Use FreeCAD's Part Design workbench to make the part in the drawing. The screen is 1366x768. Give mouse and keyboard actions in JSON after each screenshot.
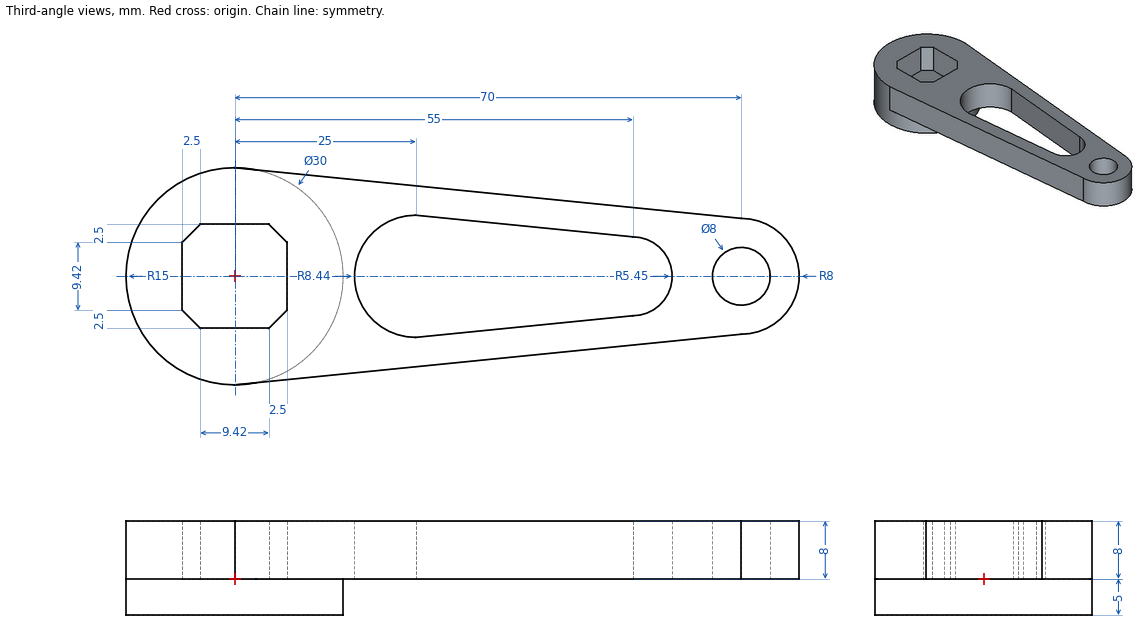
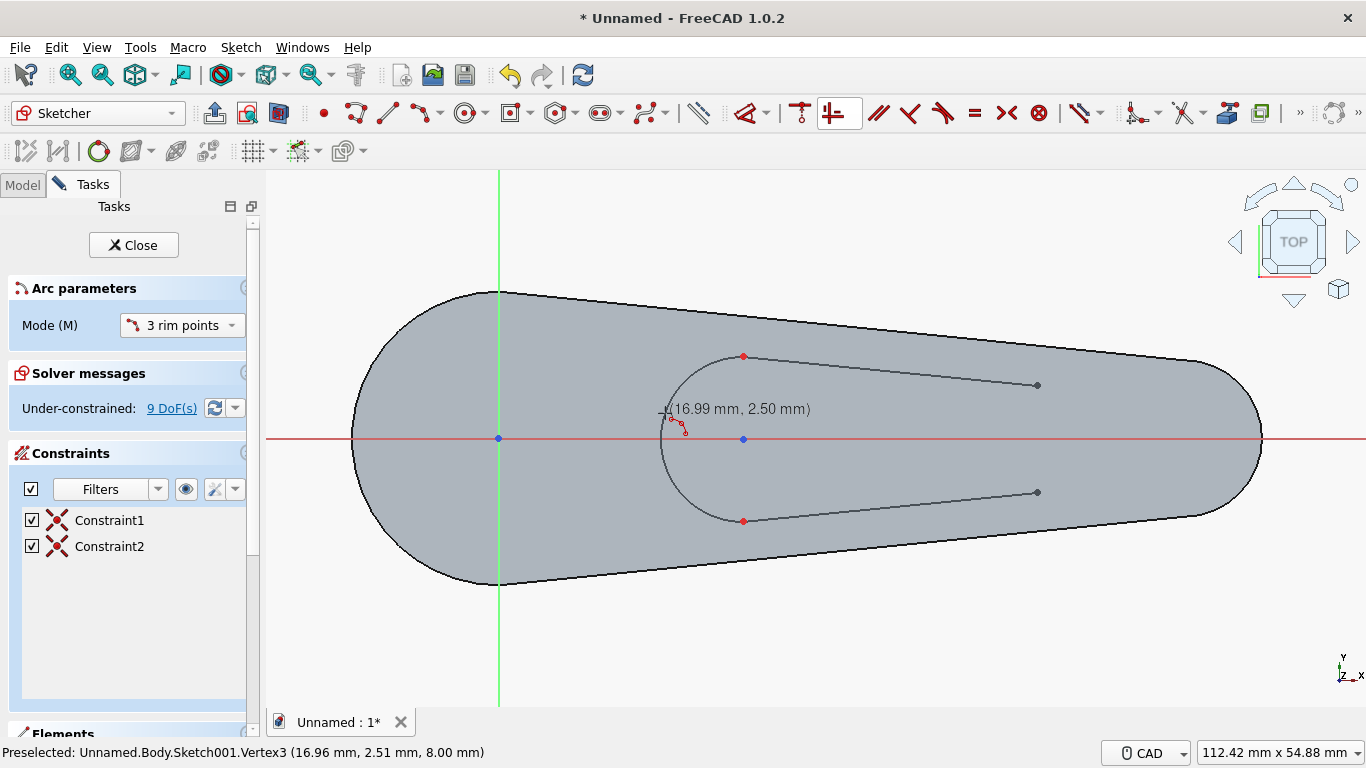
{"action": "left_click", "coordinate": [1037, 493]}
{"action": "left_click", "coordinate": [1037, 386]}
{"action": "left_click", "coordinate": [1088, 455]}
{"action": "key", "text": "Escape"}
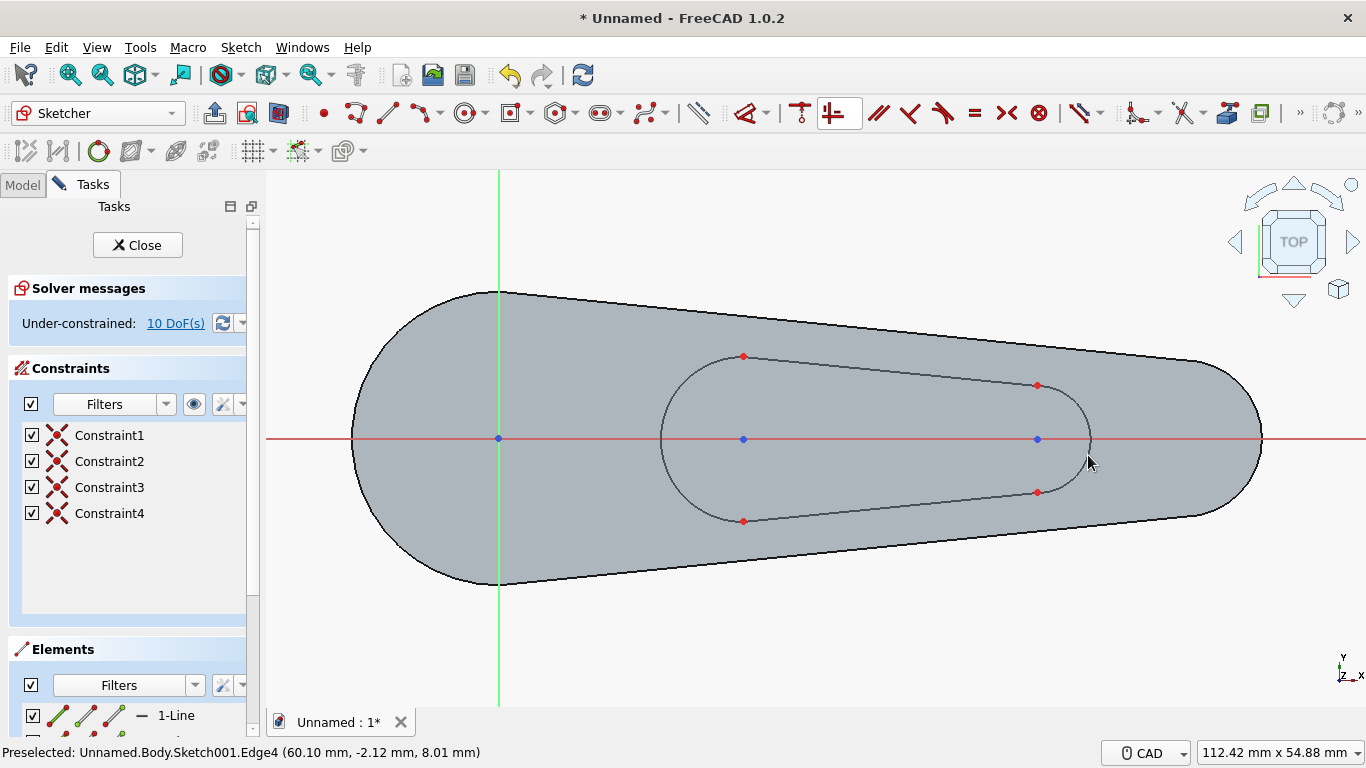
{"action": "left_click", "coordinate": [743, 439]}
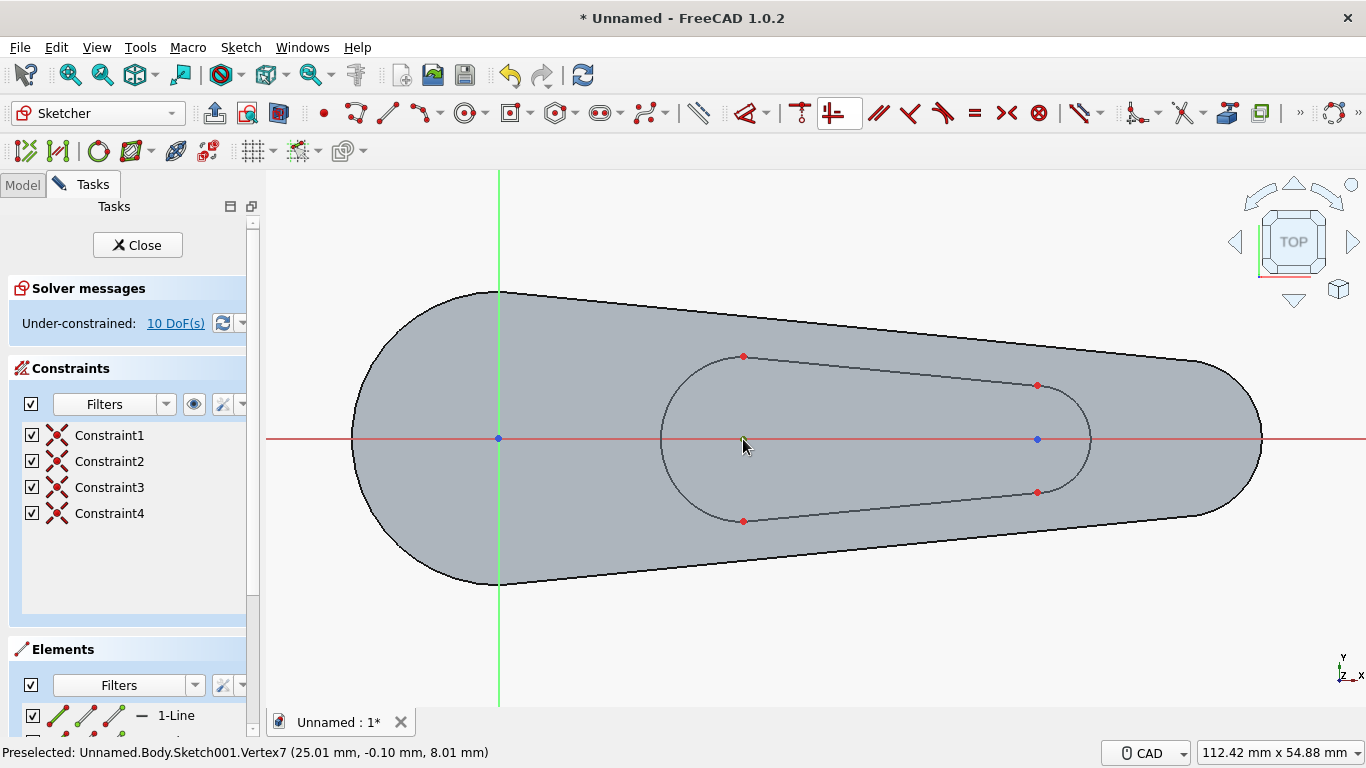
{"action": "left_click", "coordinate": [359, 438]}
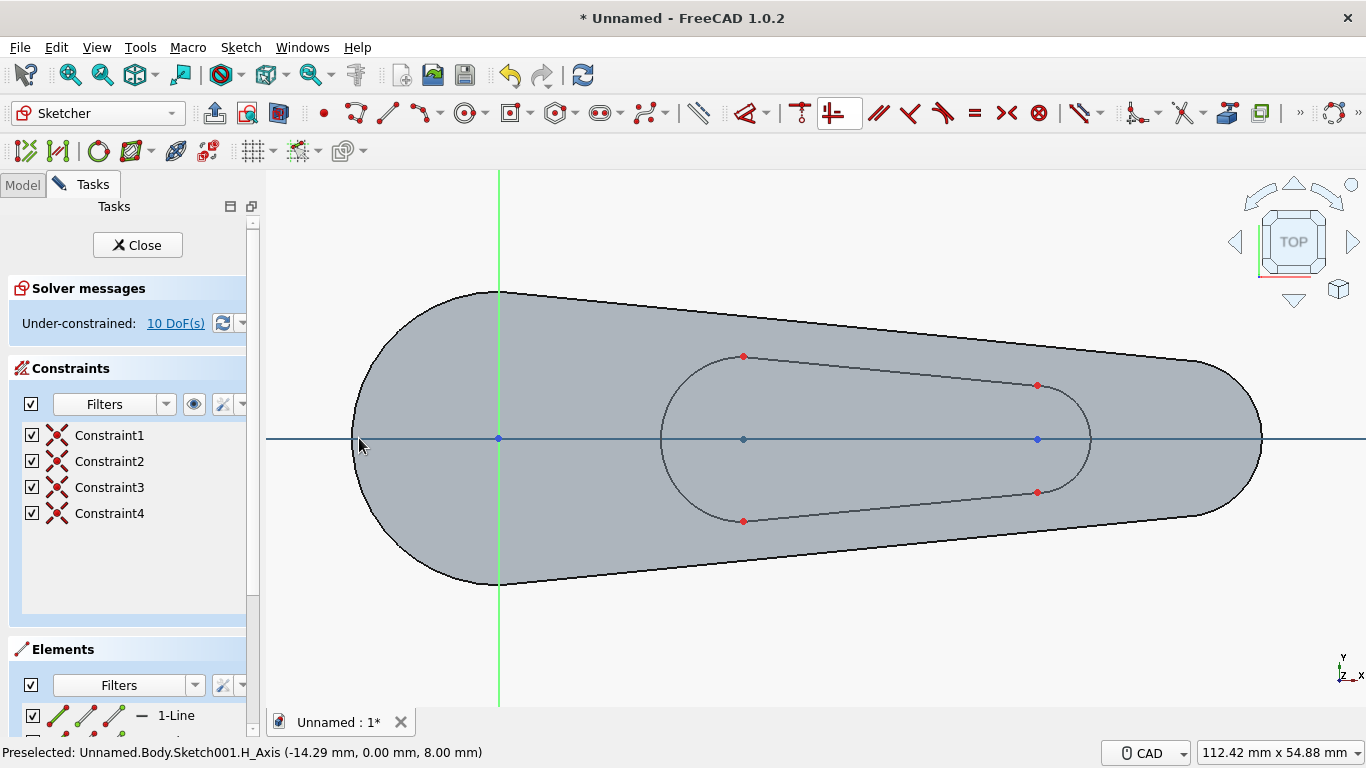
{"action": "left_click", "coordinate": [800, 114]}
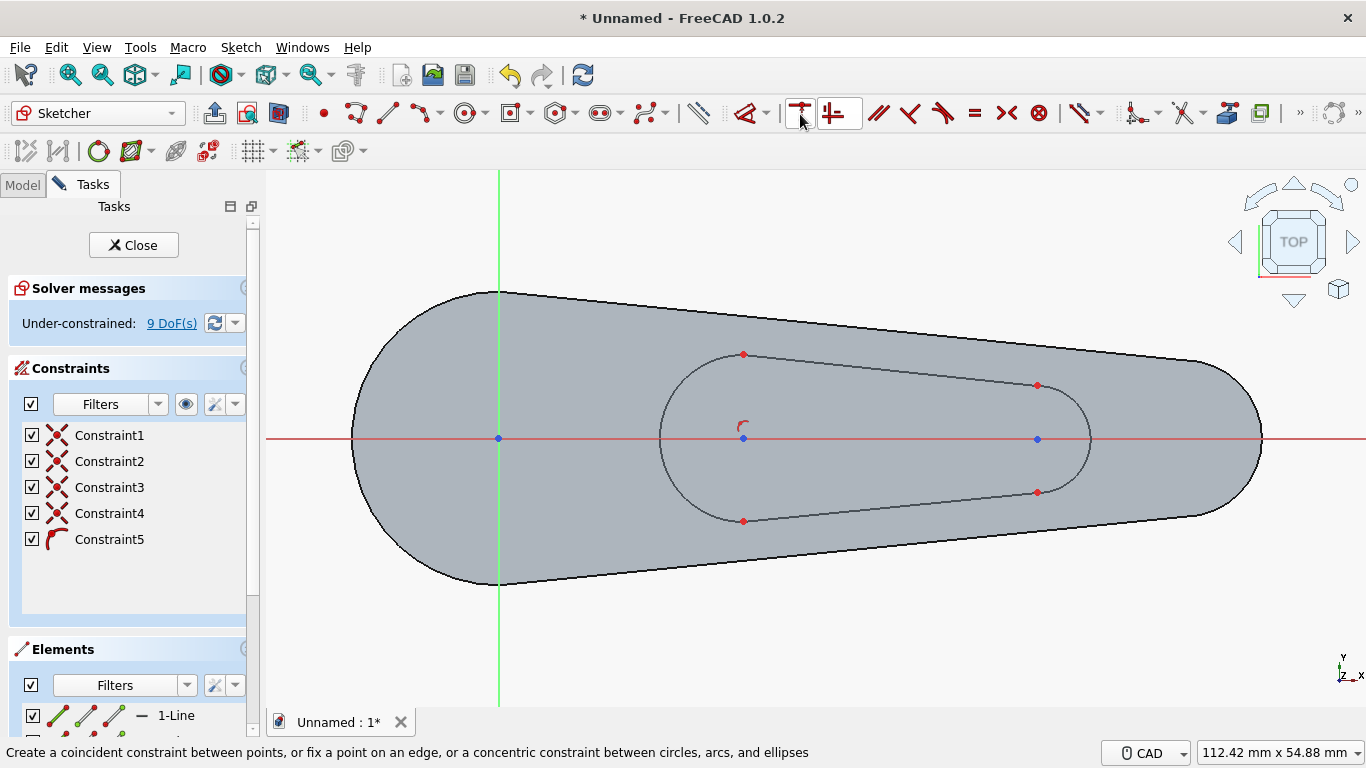
{"action": "left_click", "coordinate": [1037, 439]}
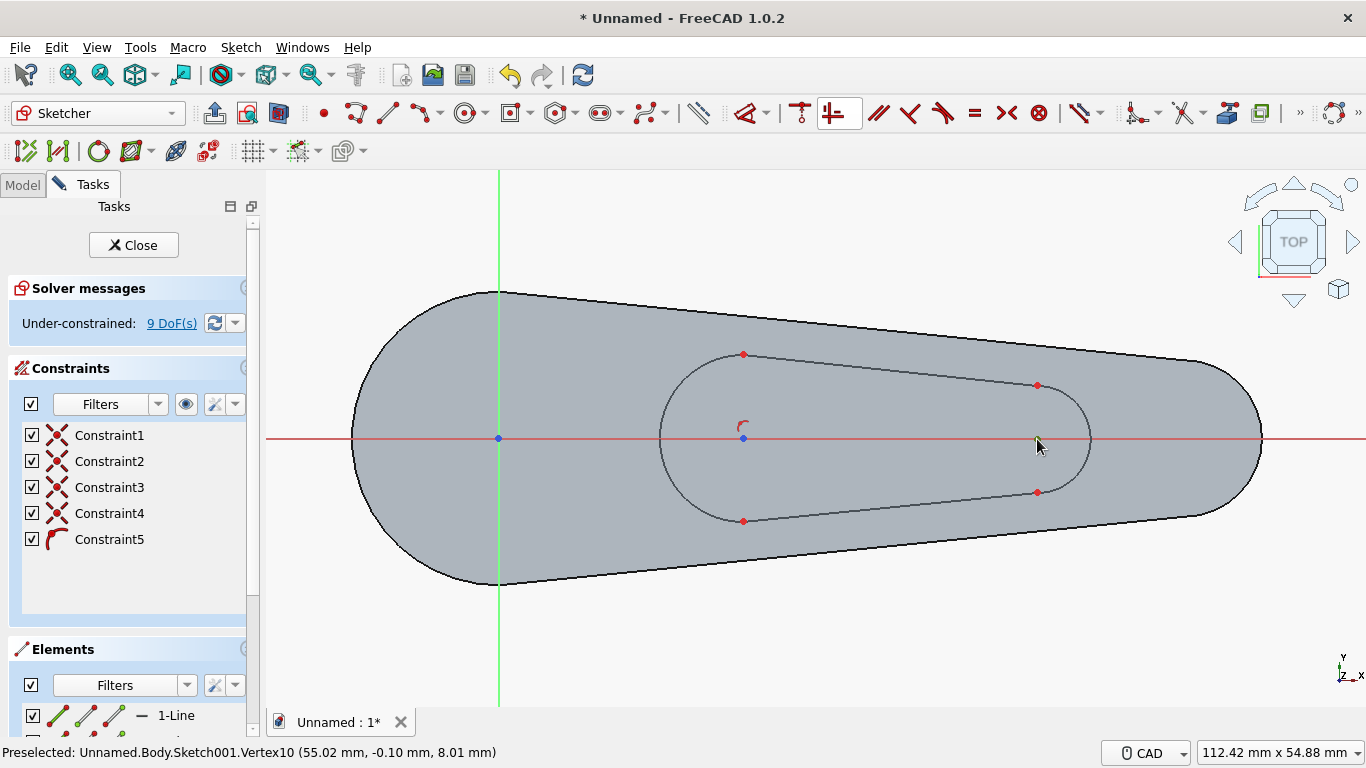
{"action": "left_click", "coordinate": [359, 438]}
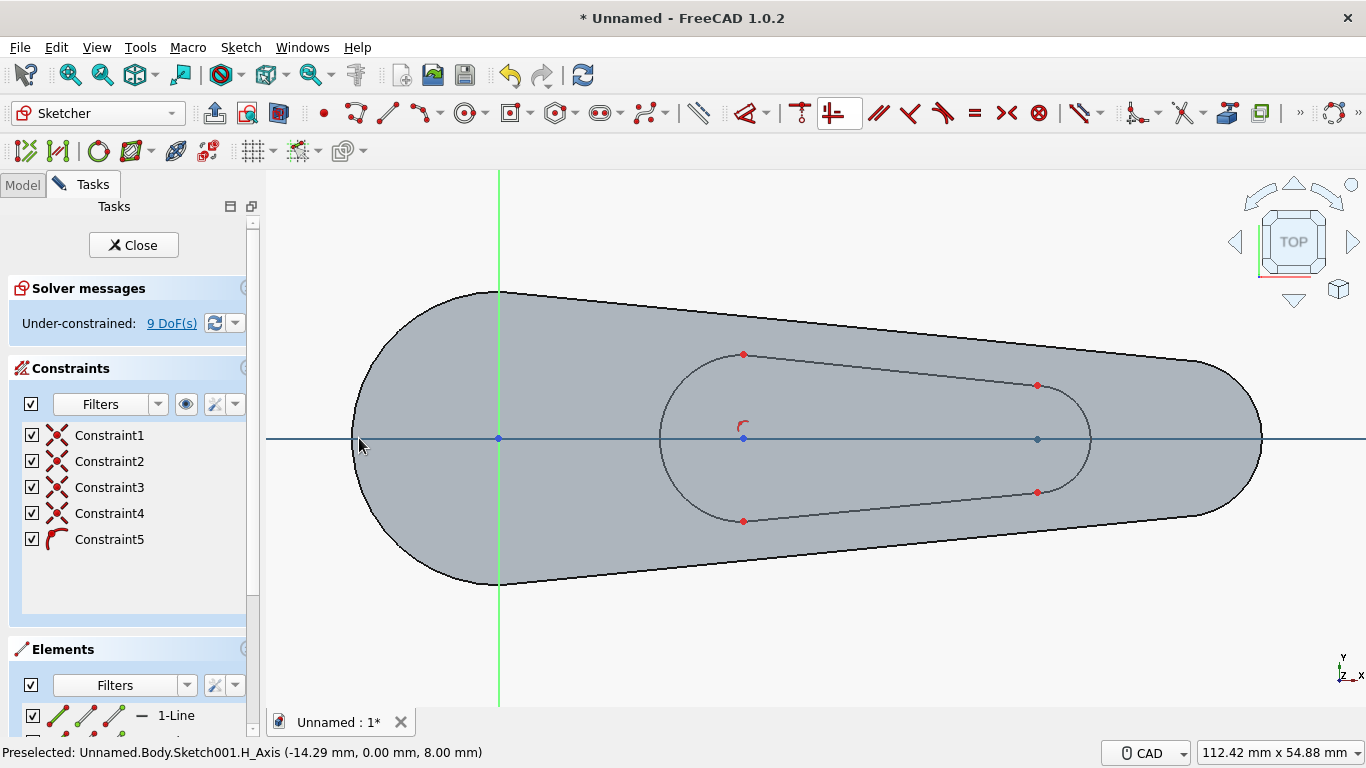
{"action": "left_click", "coordinate": [800, 114]}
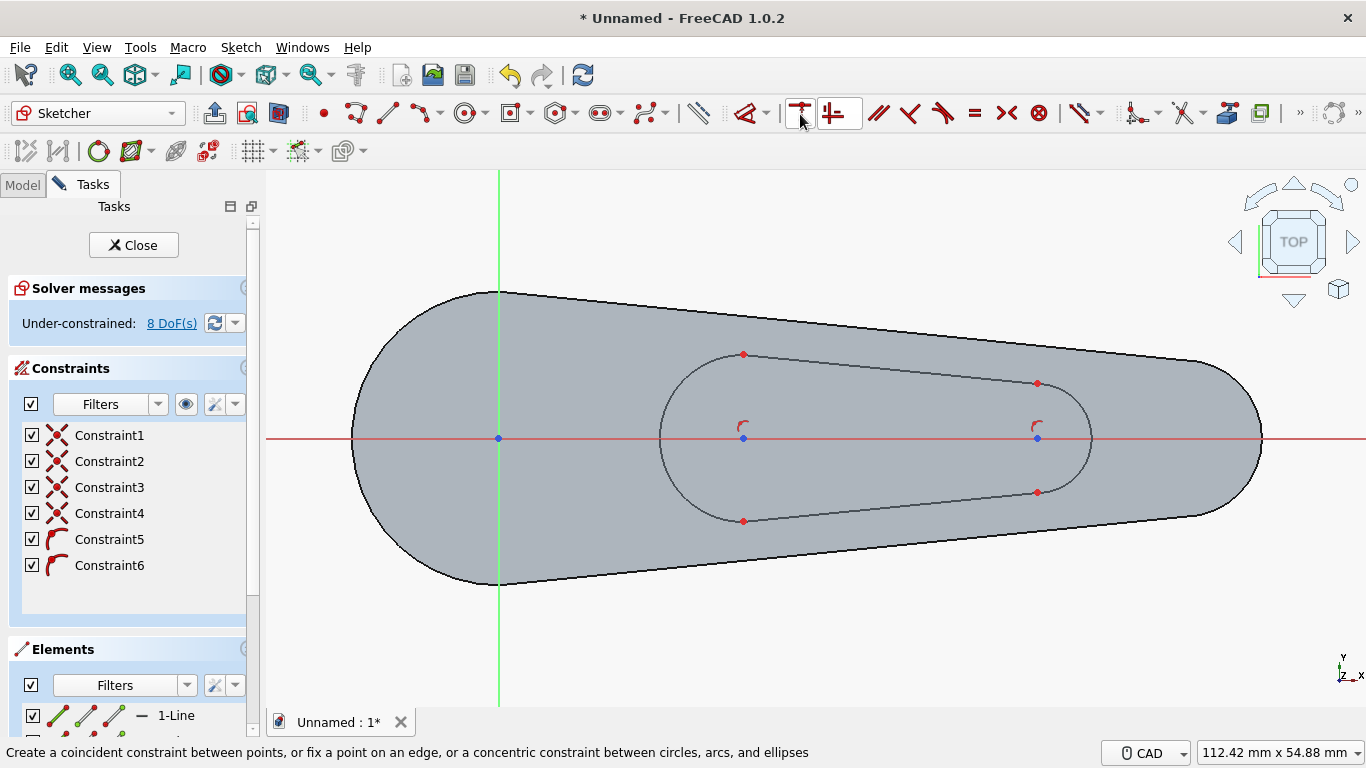
{"action": "left_click", "coordinate": [746, 114]}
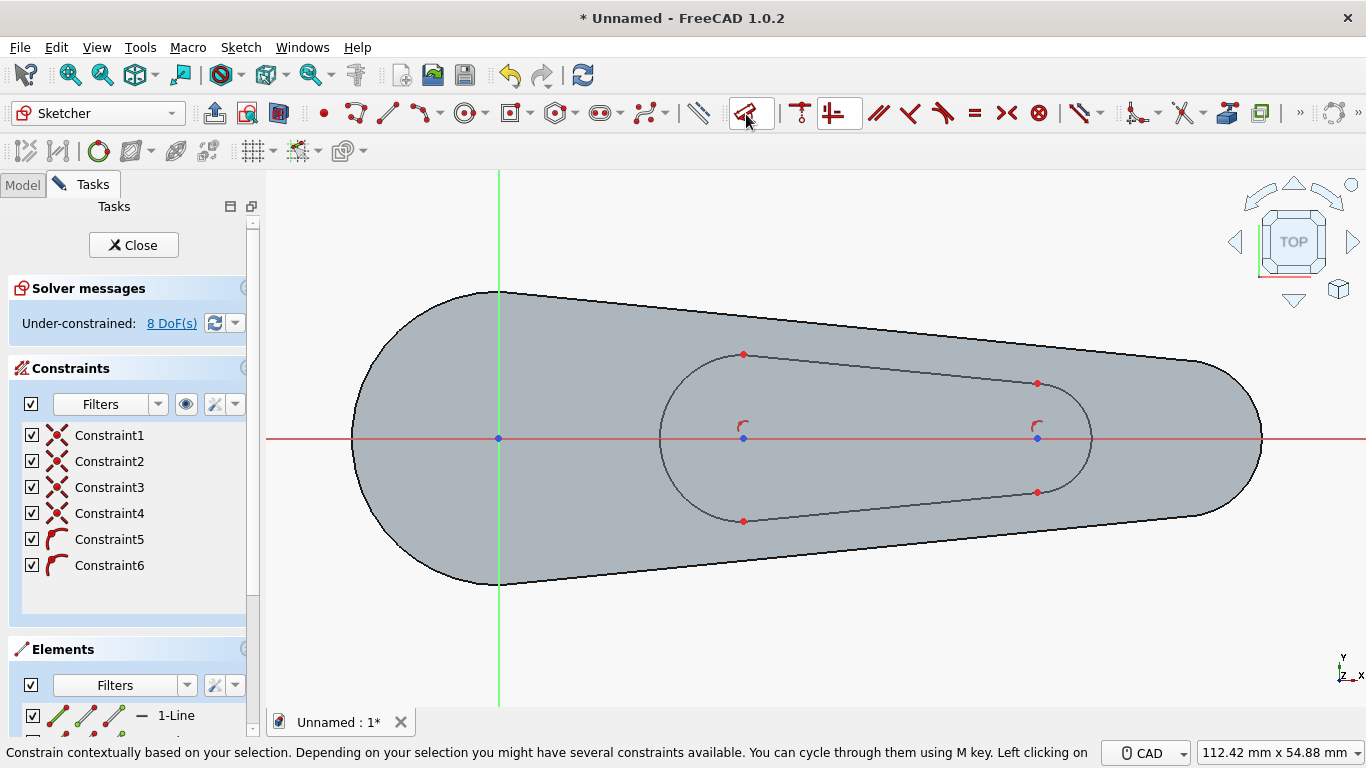
{"action": "left_click", "coordinate": [676, 390]}
{"action": "left_click", "coordinate": [650, 371]}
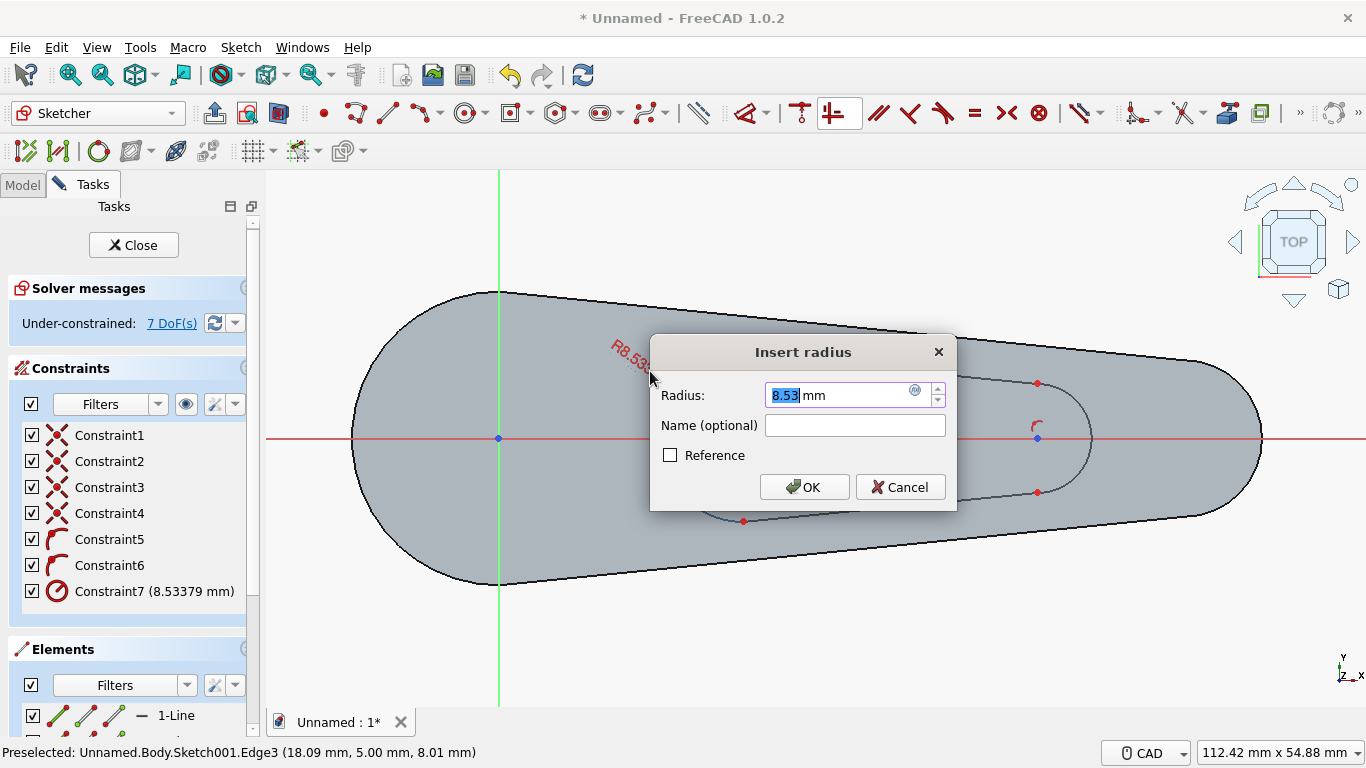
{"action": "type", "text": "8.44"}
{"action": "key", "text": "Return"}